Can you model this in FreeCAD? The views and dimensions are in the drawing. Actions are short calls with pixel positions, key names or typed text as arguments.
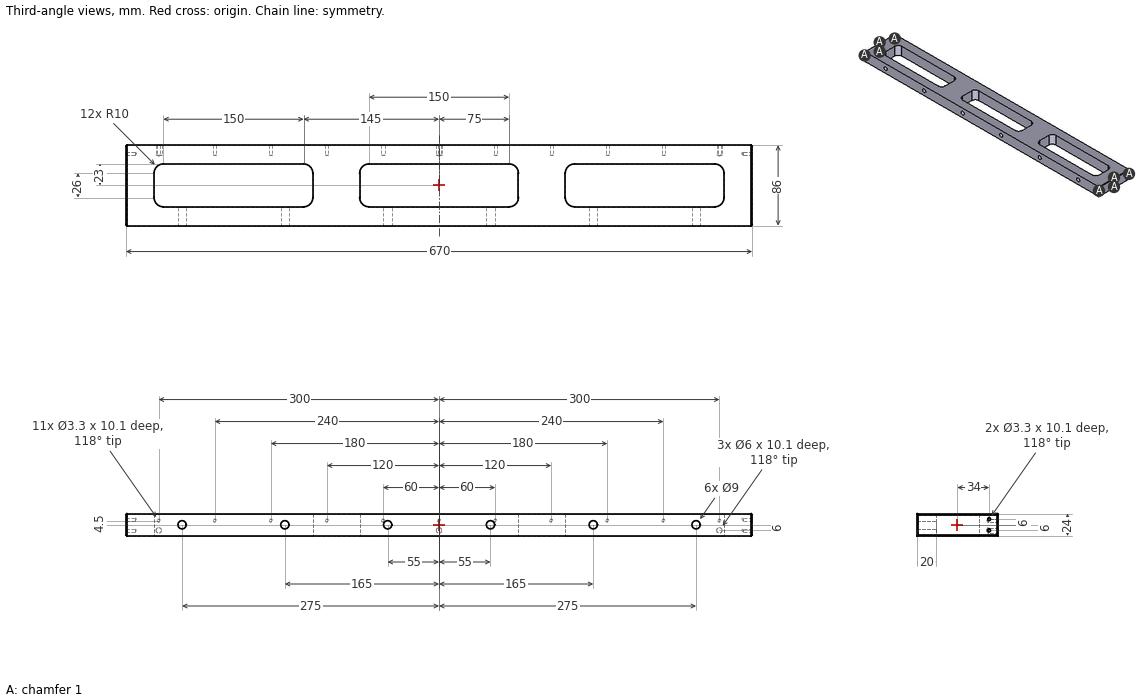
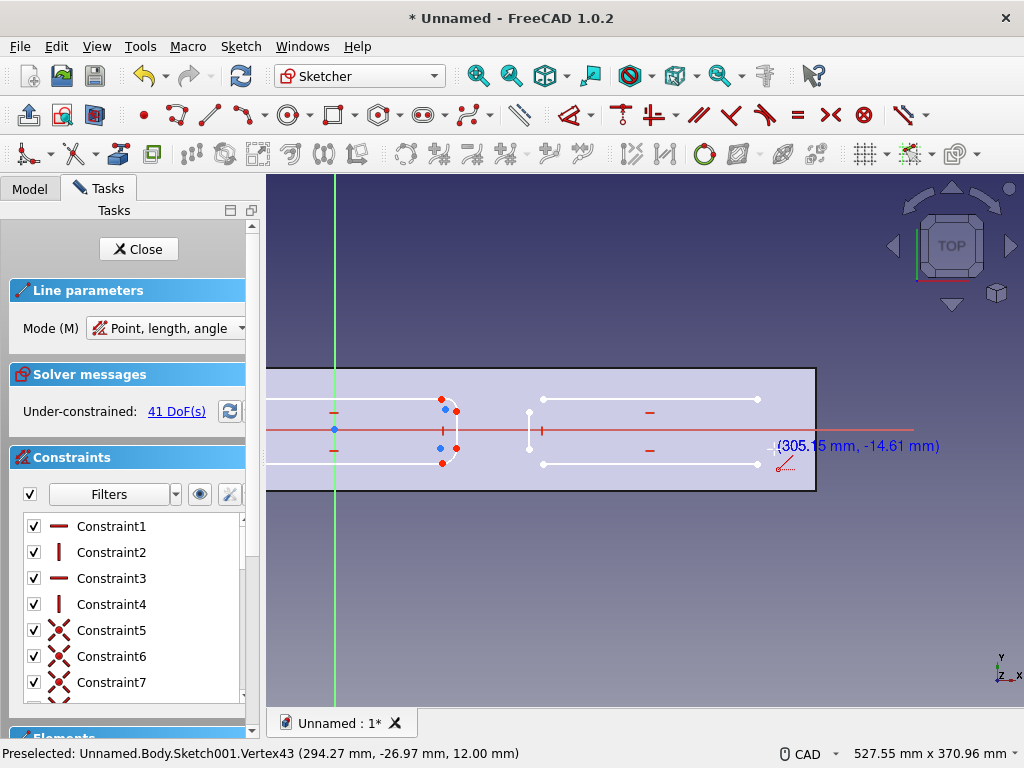
click(773, 448)
click(773, 411)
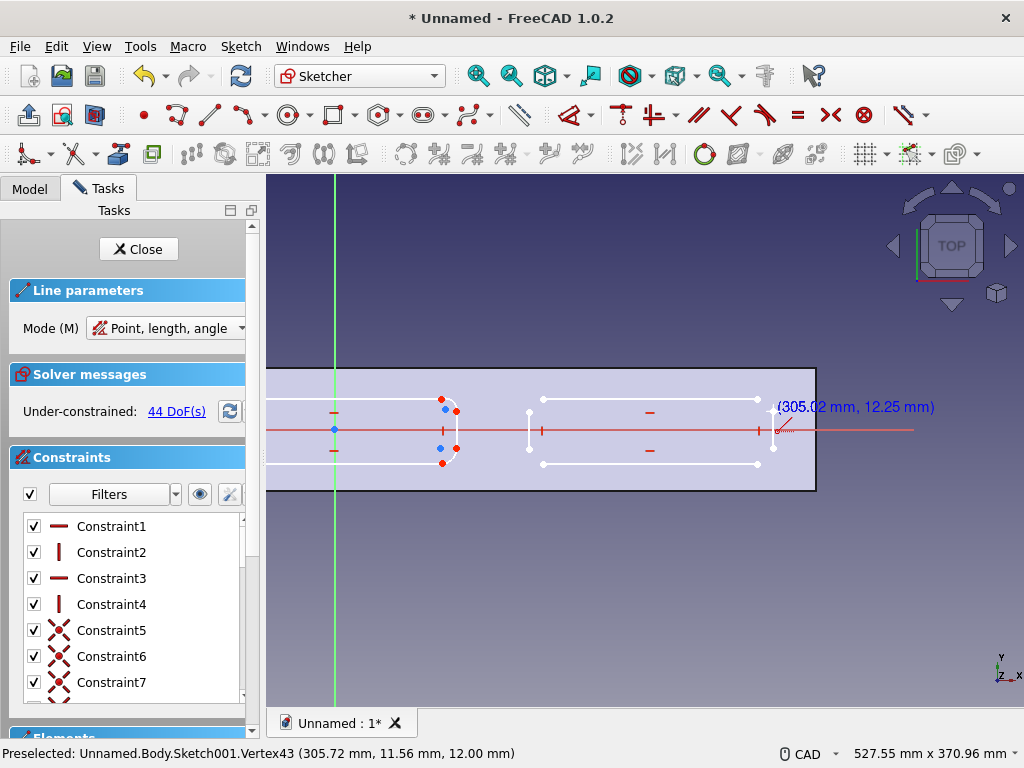
key(g)
key(3)
key(a)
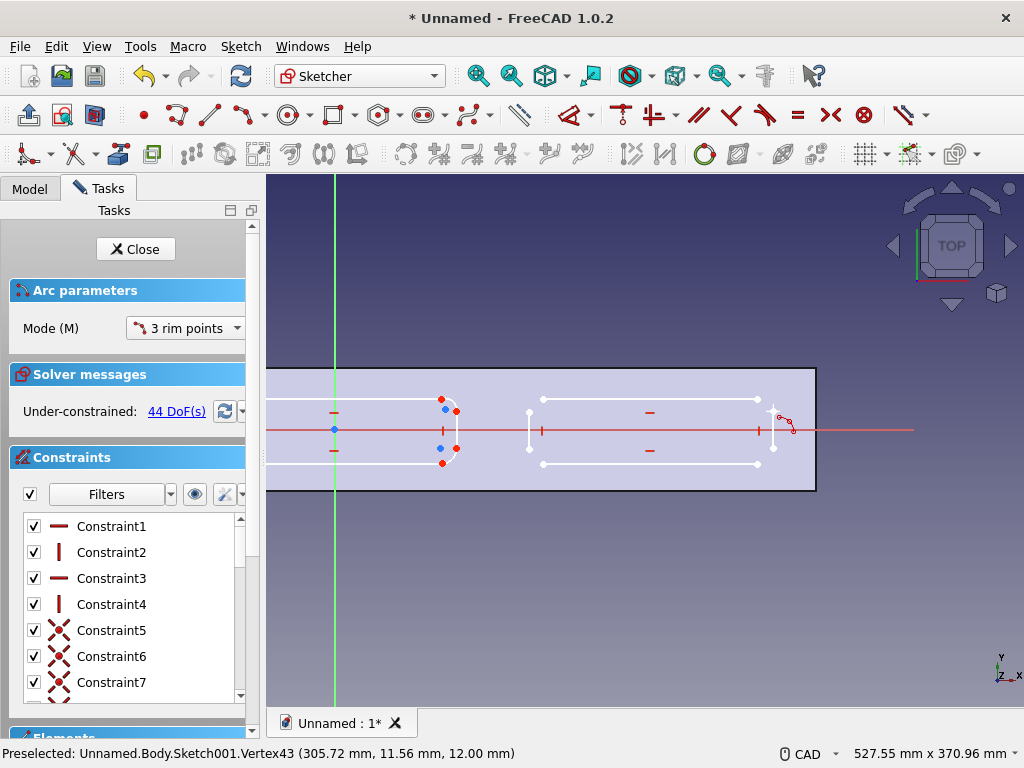
click(544, 399)
click(529, 412)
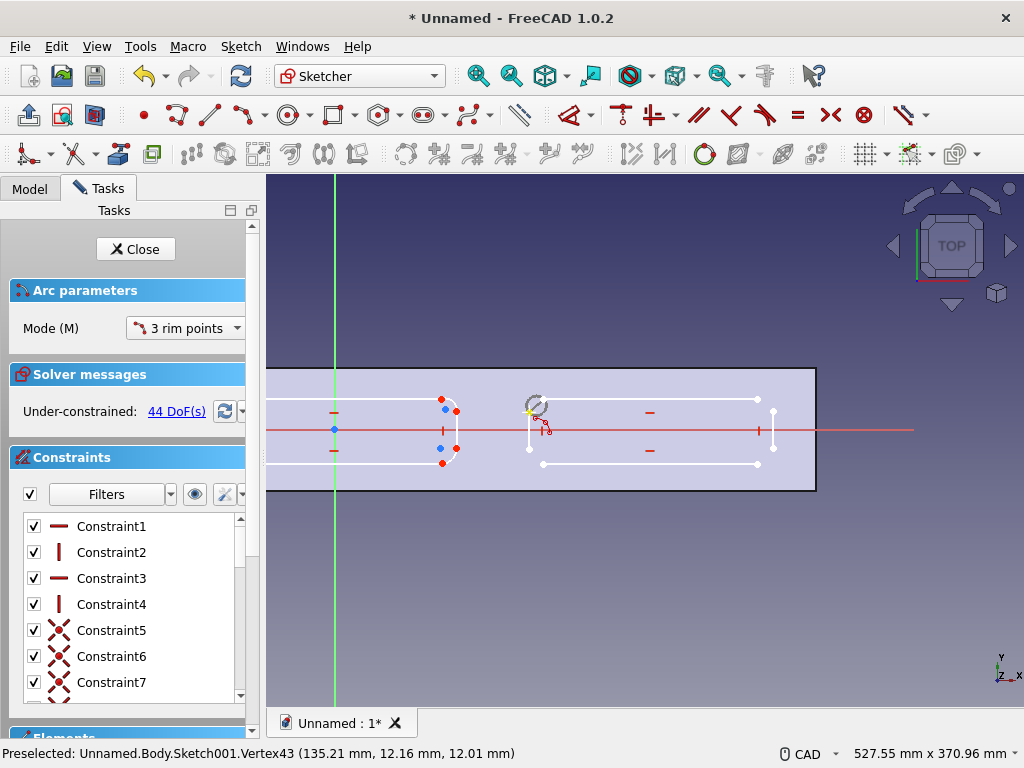
scroll(533, 401, up, 7)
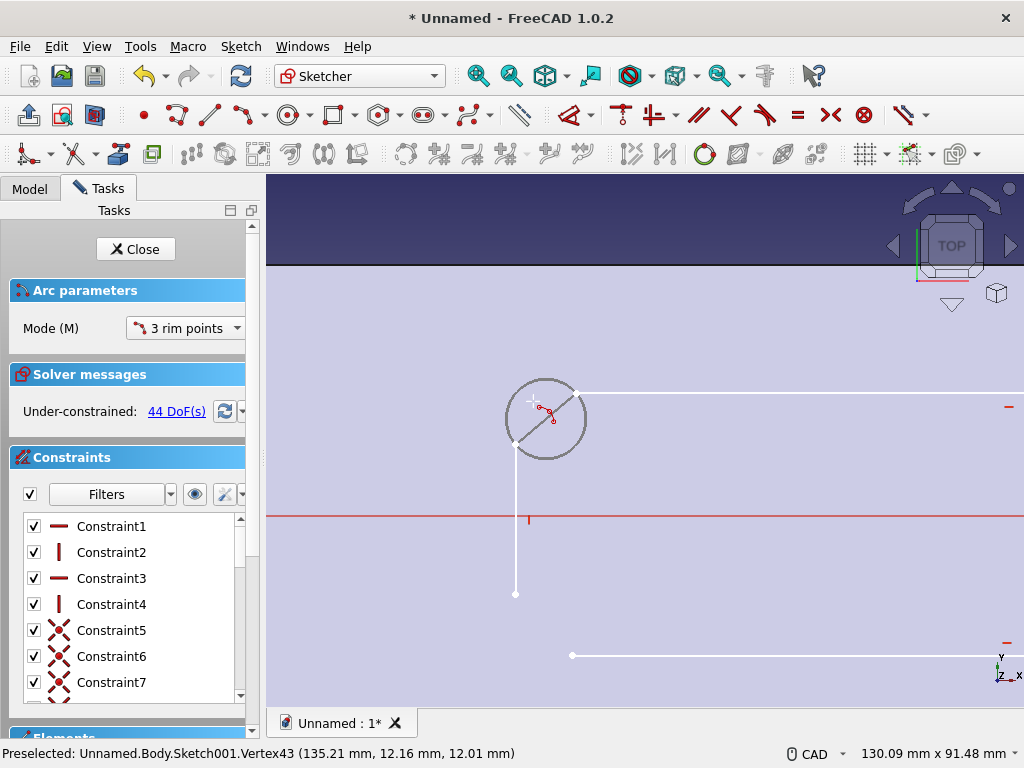
click(532, 399)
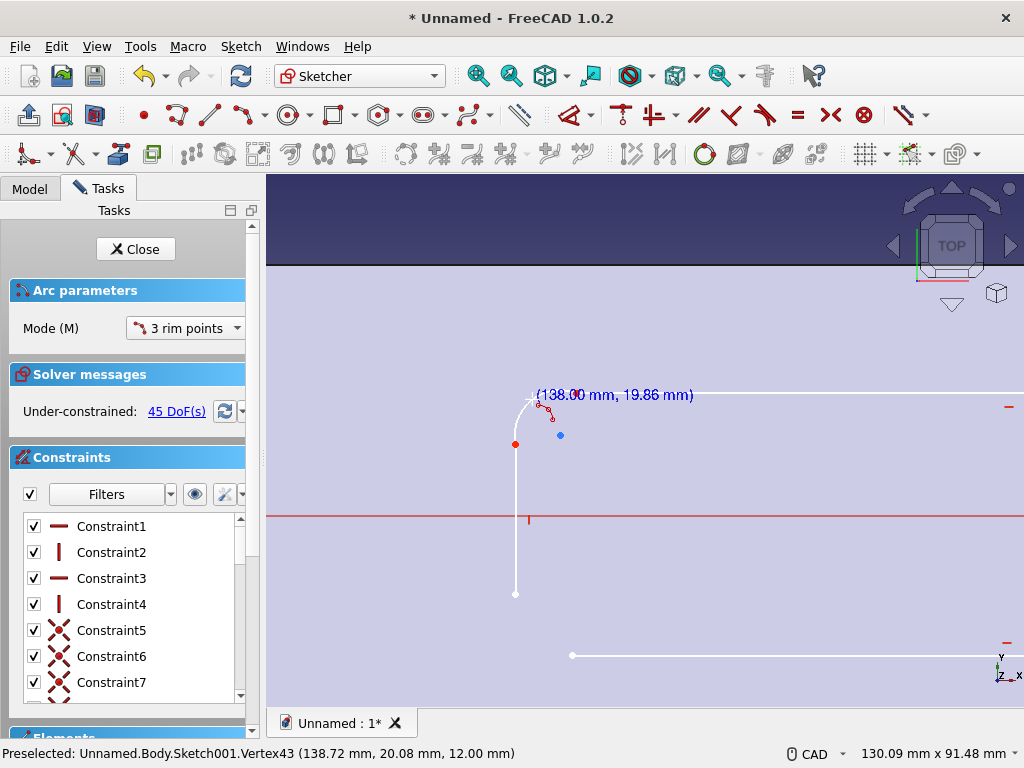
scroll(682, 431, down, 11)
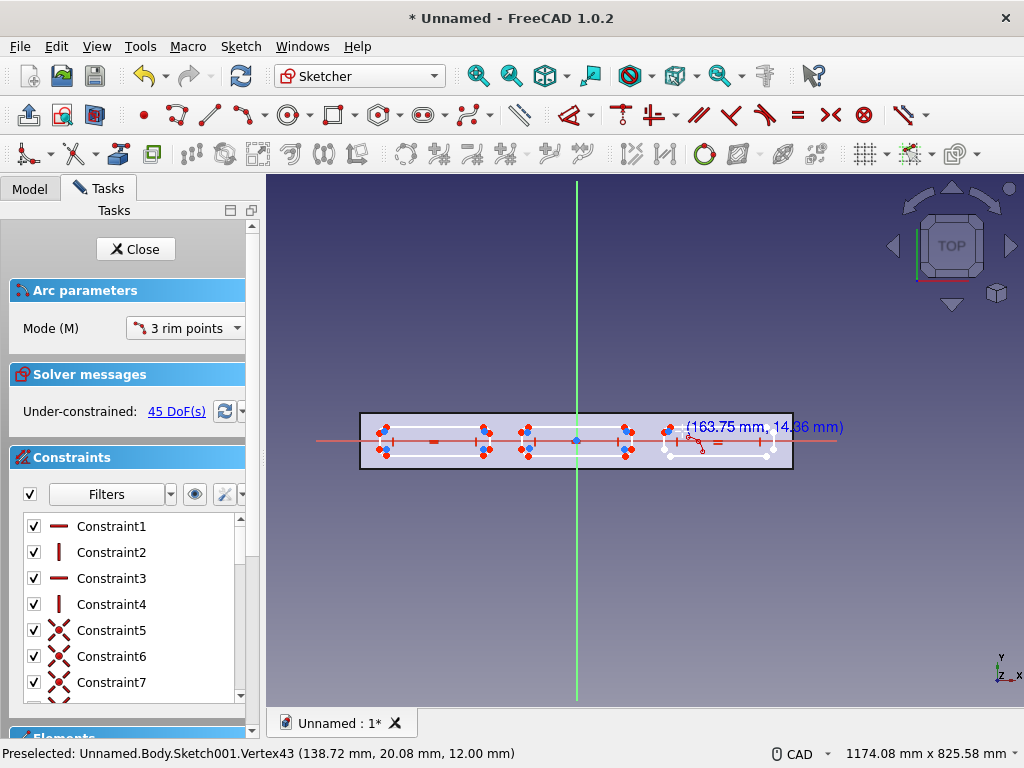
scroll(664, 449, up, 4)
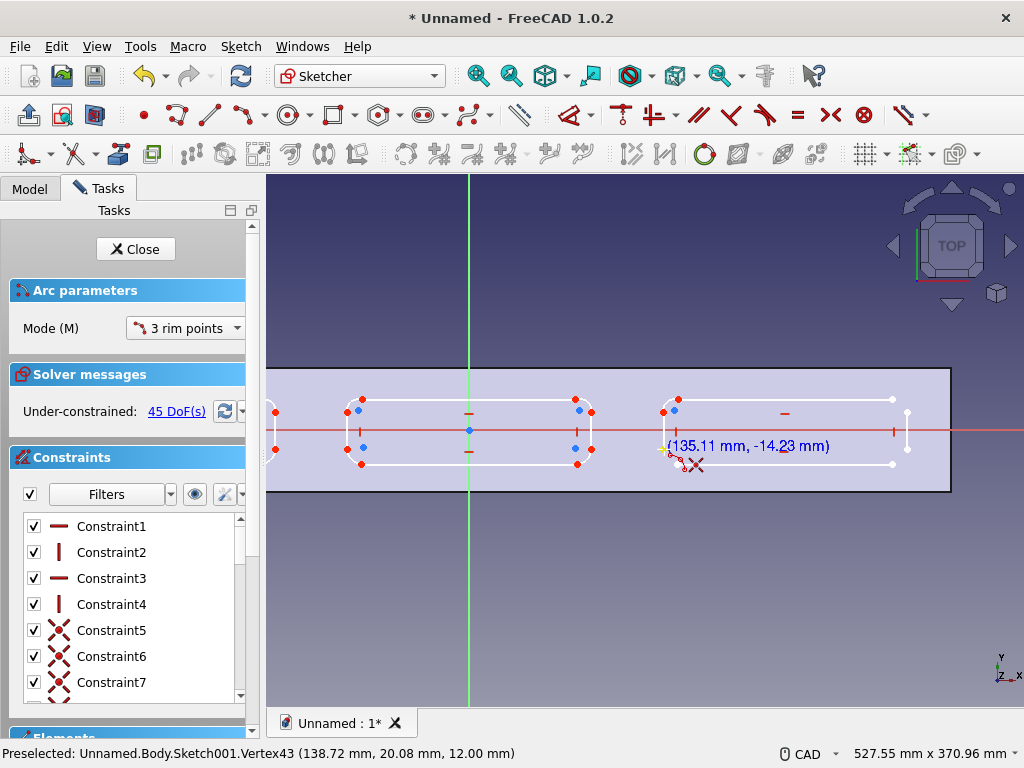
click(664, 450)
click(678, 465)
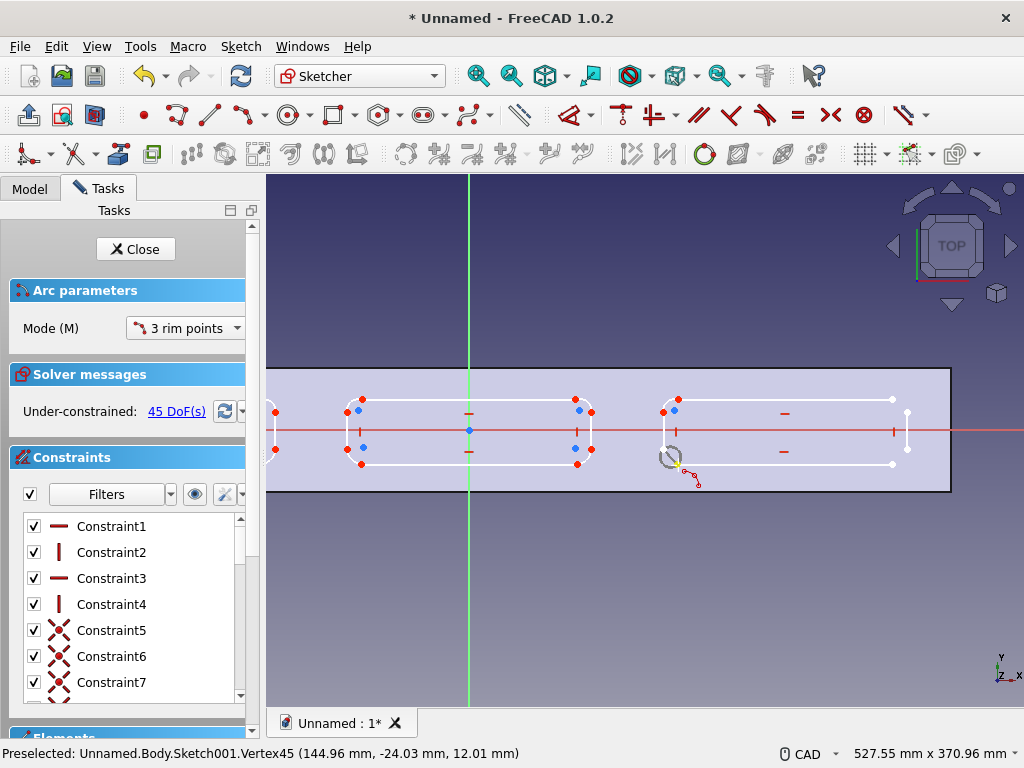
scroll(667, 459, up, 7)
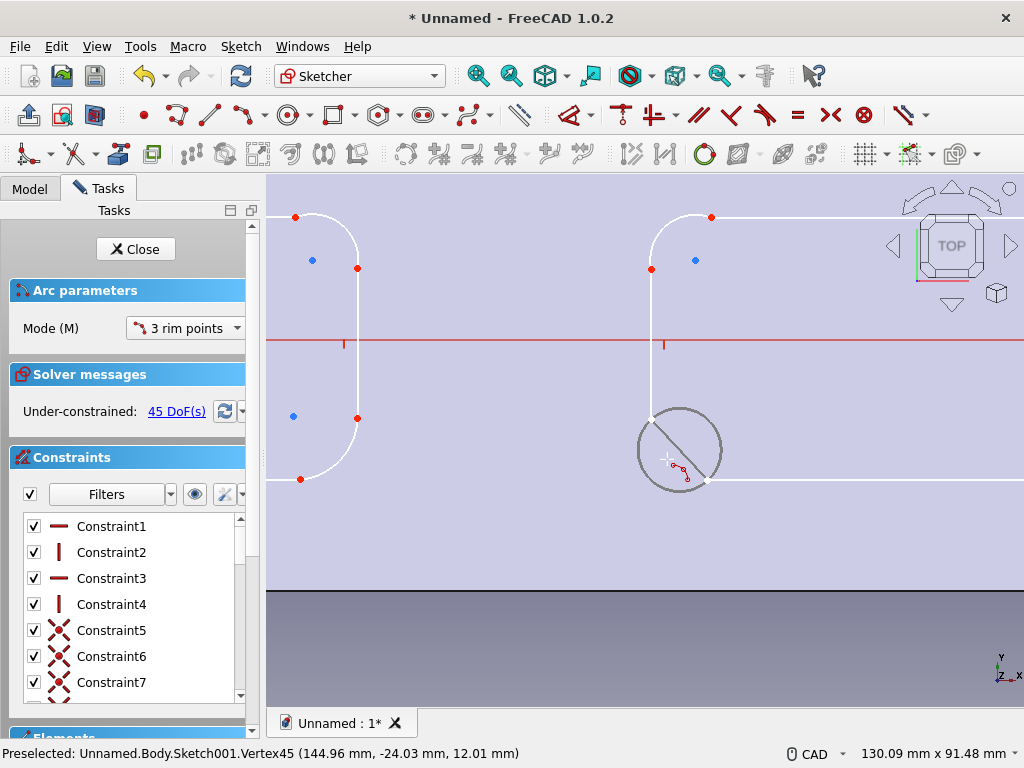
click(667, 457)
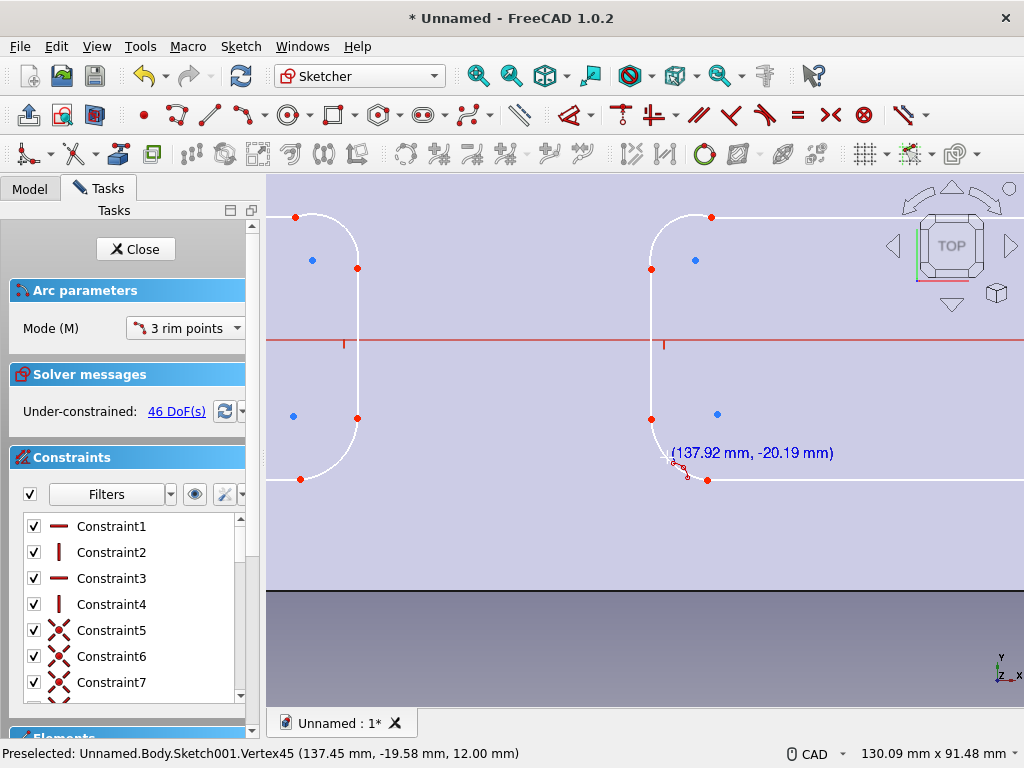
scroll(665, 453, down, 11)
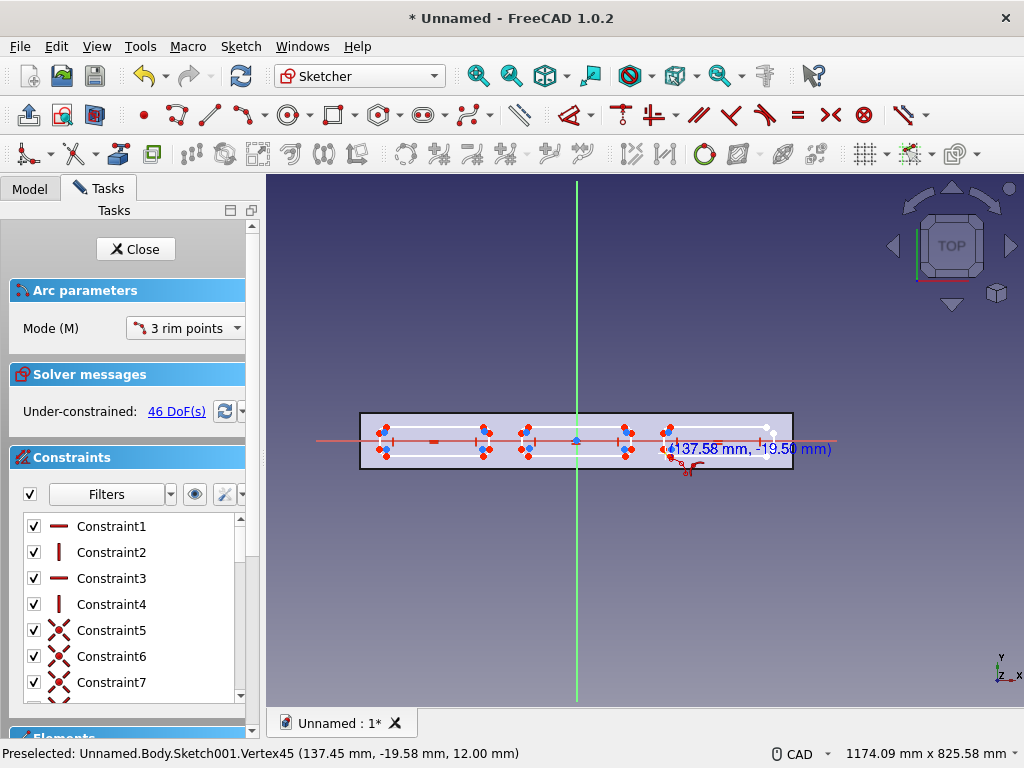
scroll(767, 456, up, 3)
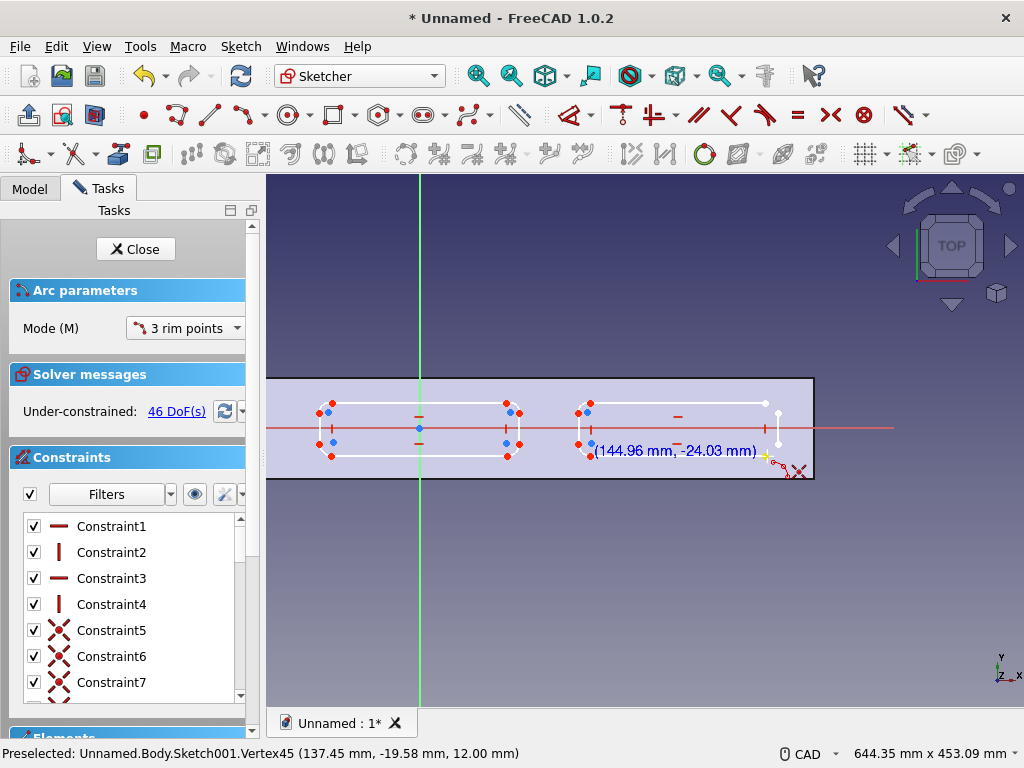
click(766, 456)
click(778, 444)